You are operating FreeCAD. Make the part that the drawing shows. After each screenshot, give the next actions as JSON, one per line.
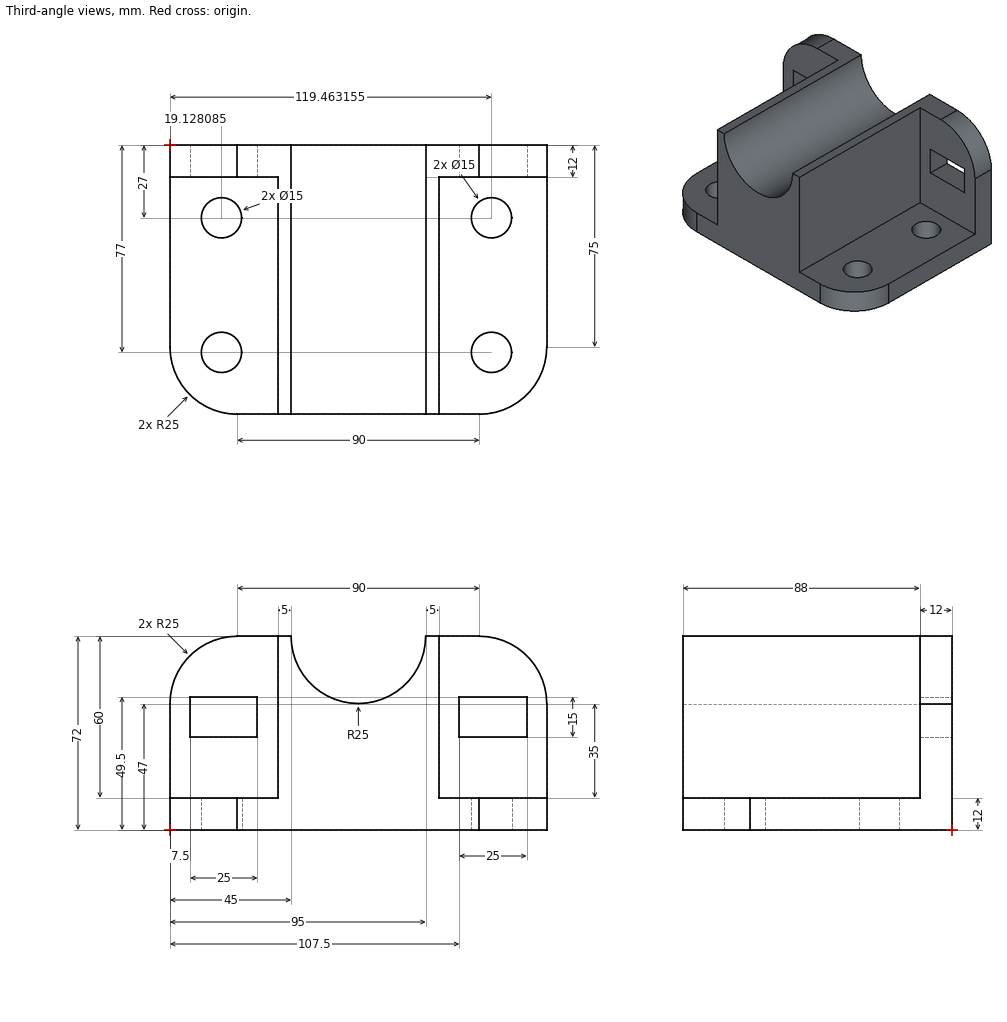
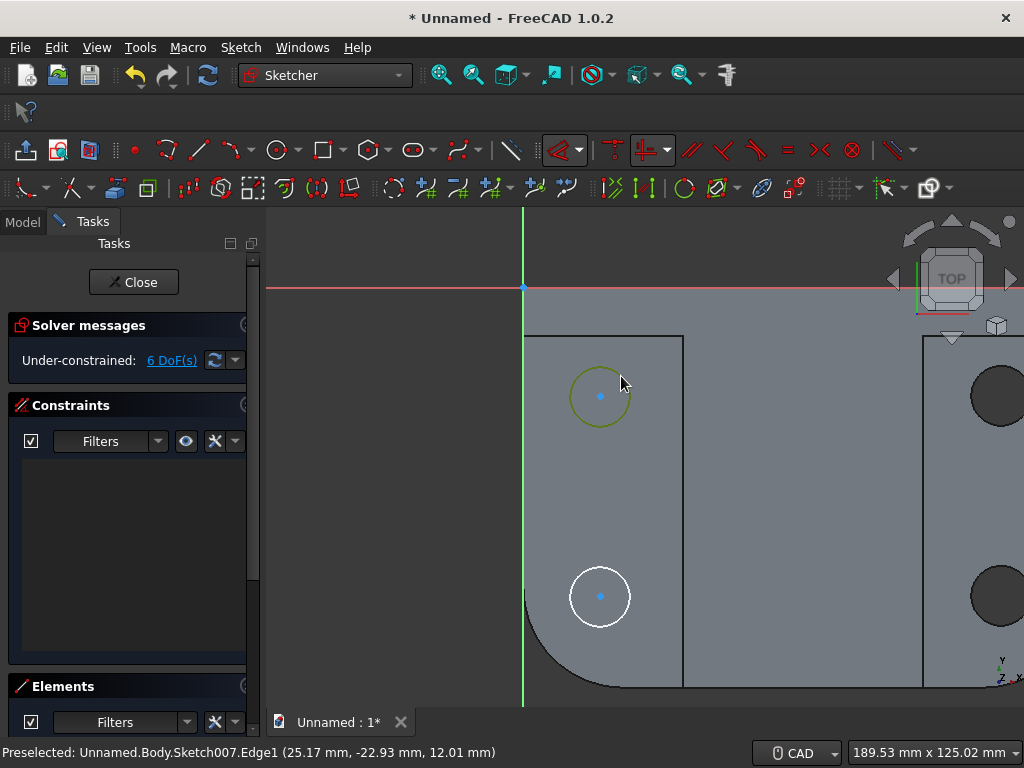
{"action": "left_click", "coordinate": [621, 576]}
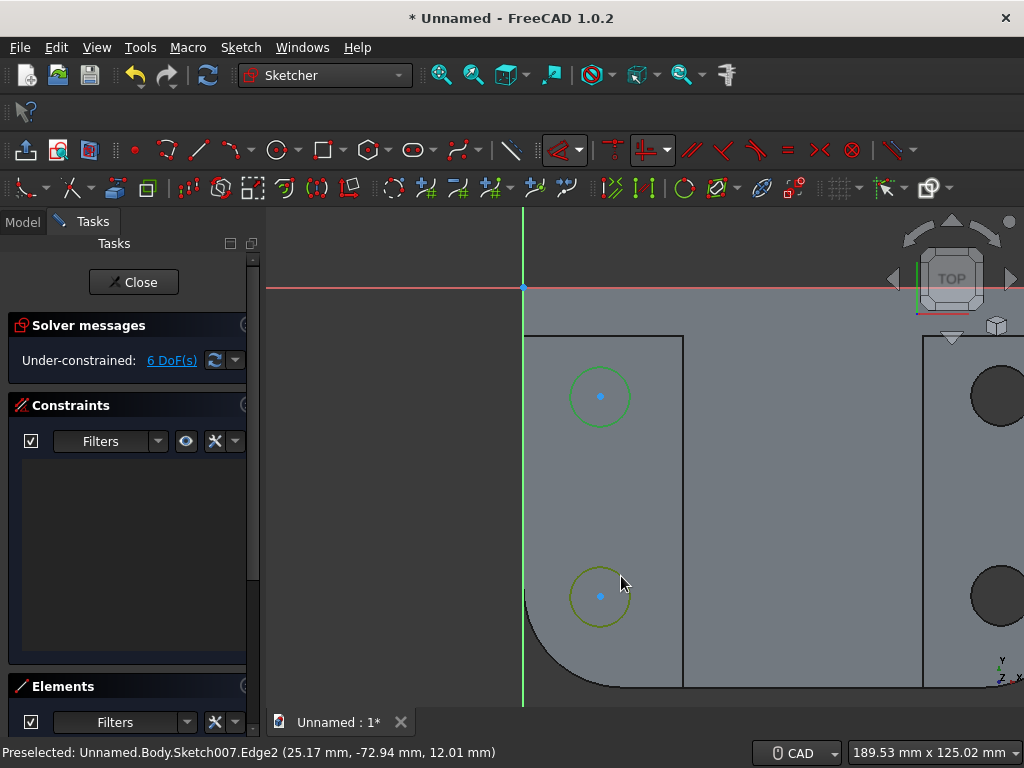
{"action": "left_click", "coordinate": [788, 150]}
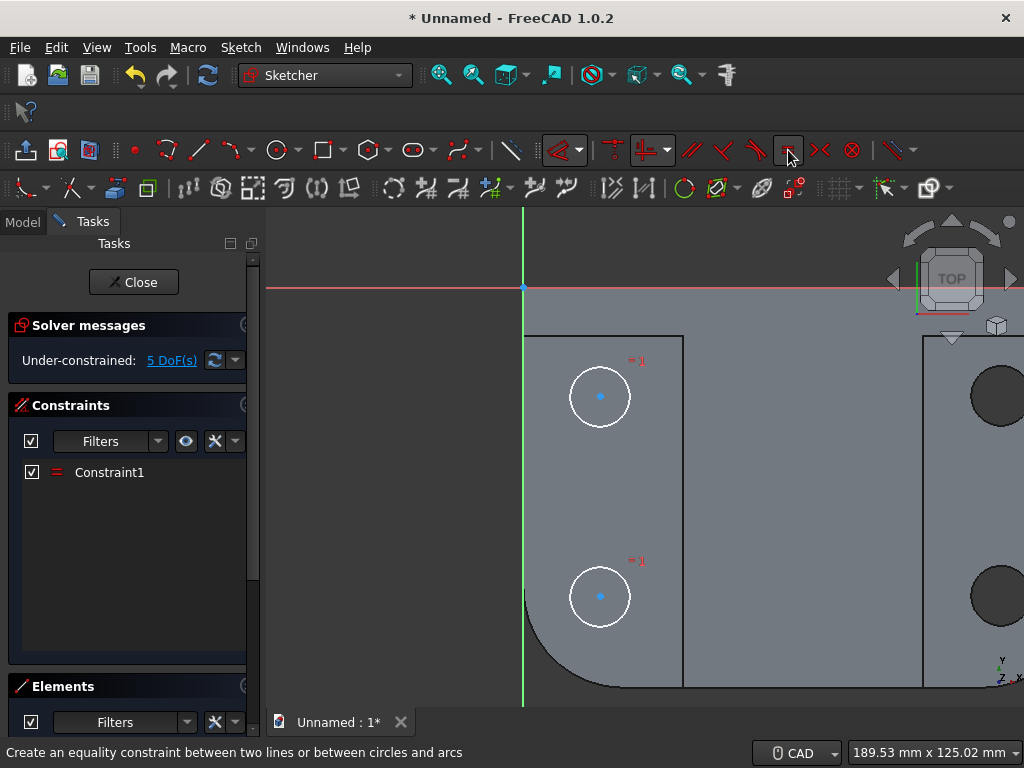
{"action": "left_click", "coordinate": [600, 397]}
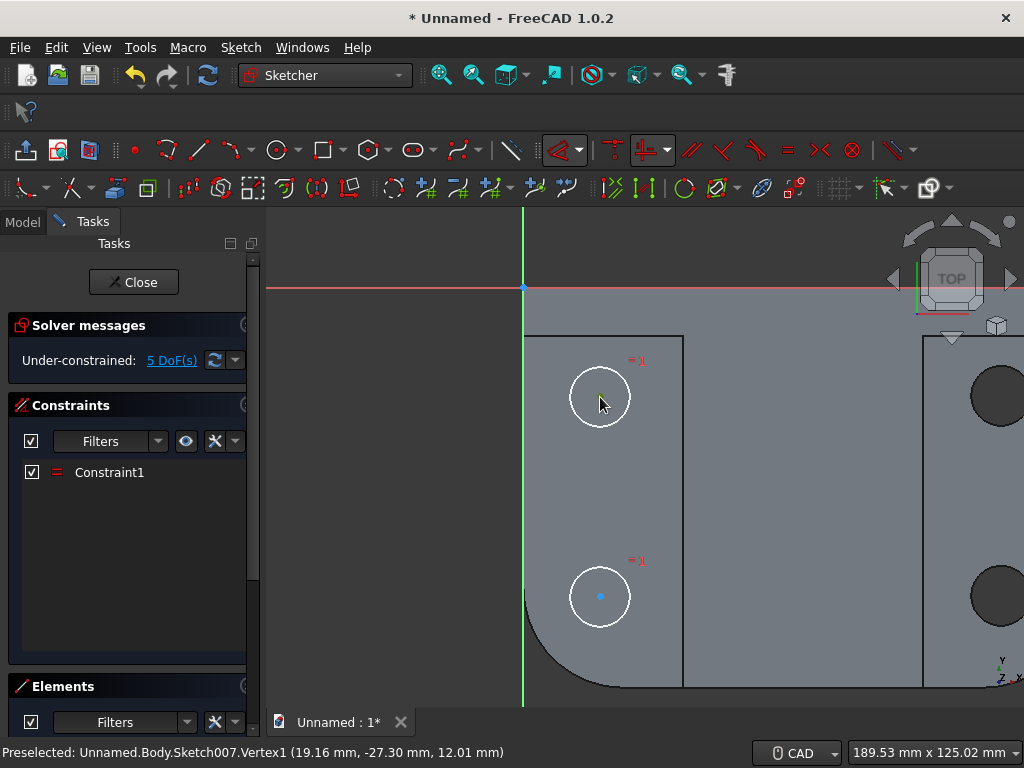
{"action": "left_click", "coordinate": [600, 597]}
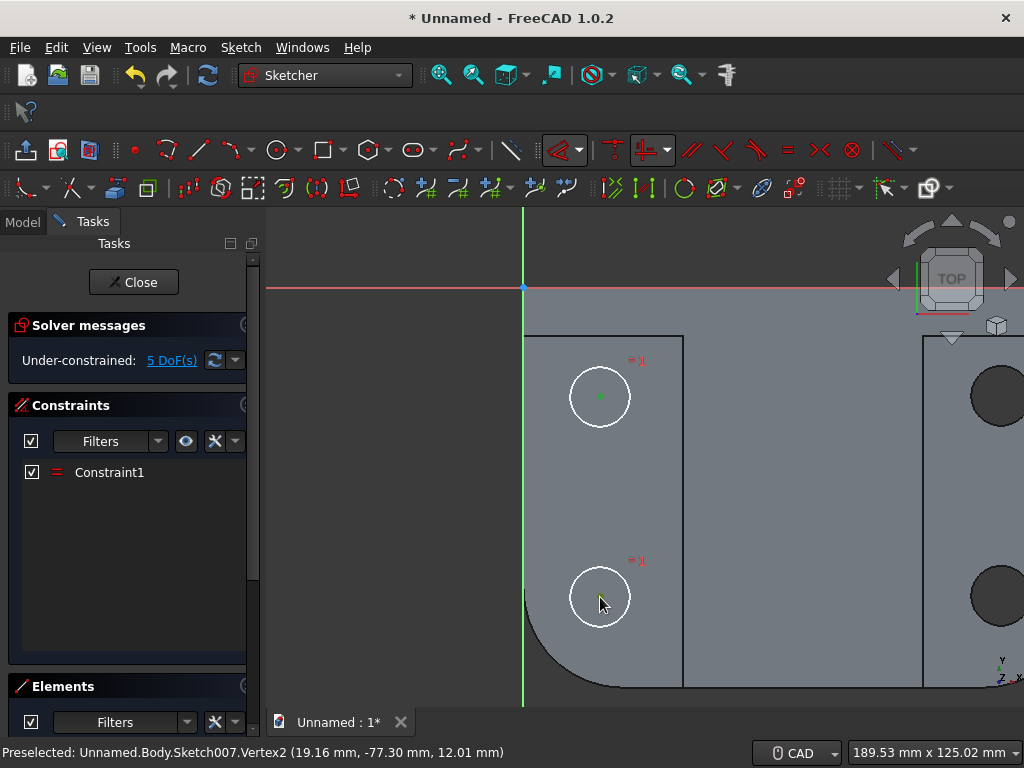
{"action": "key", "text": "v"}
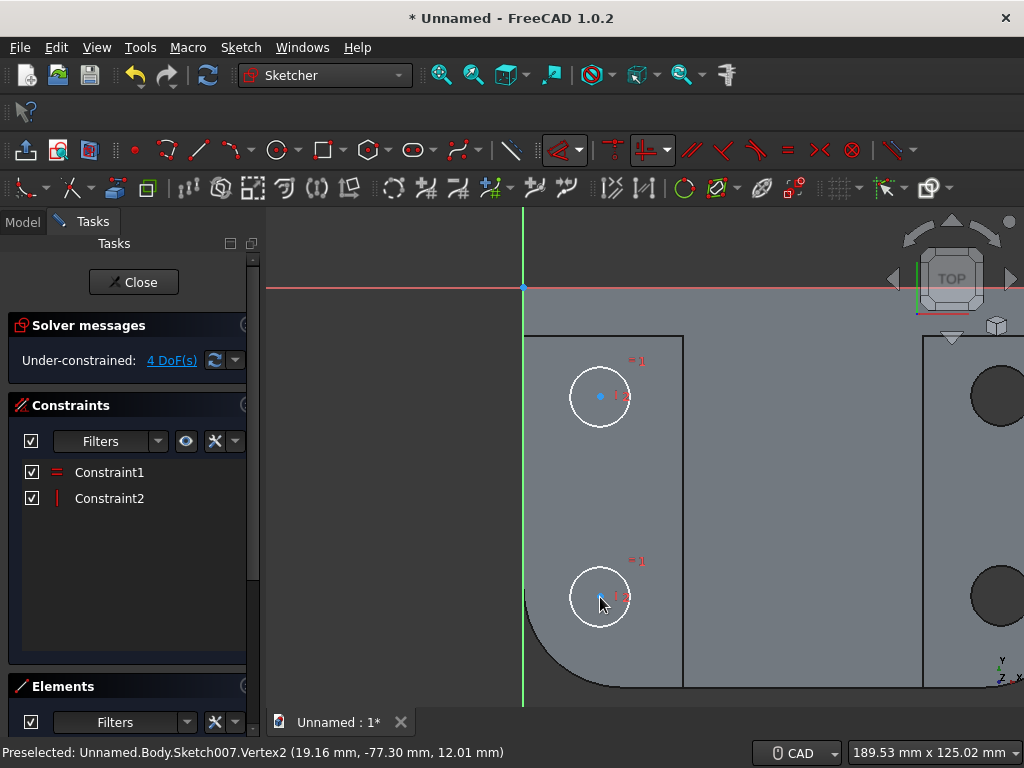
{"action": "left_click", "coordinate": [621, 376]}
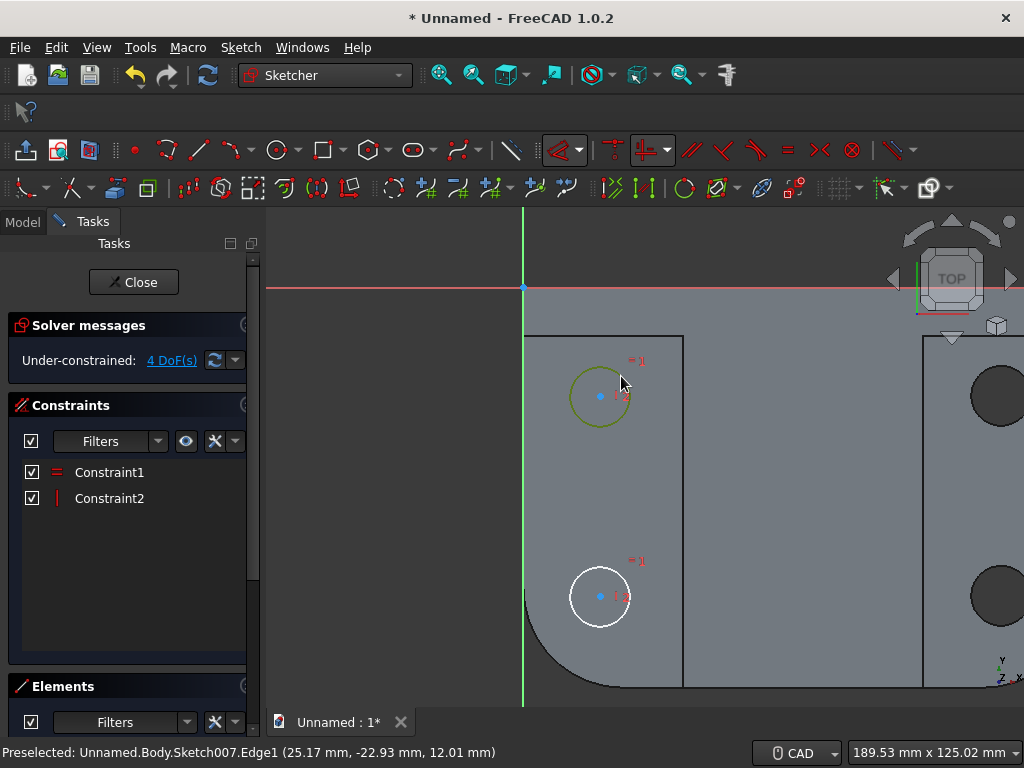
{"action": "key", "text": "k o"}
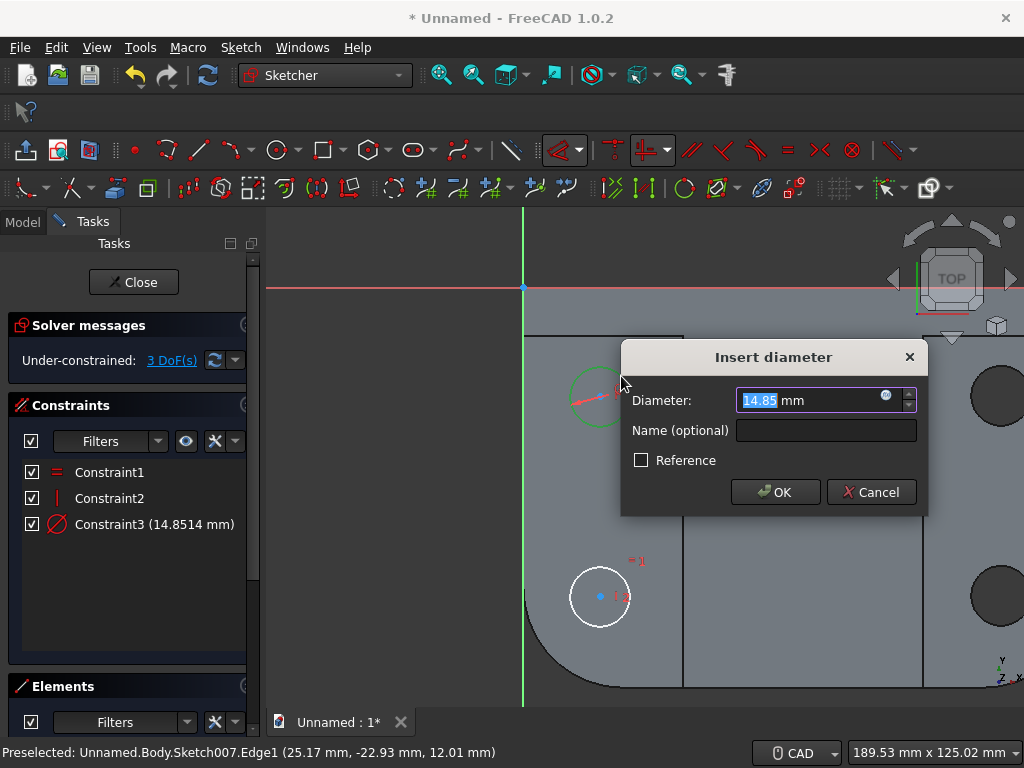
{"action": "type", "text": "15"}
{"action": "key", "text": "Return"}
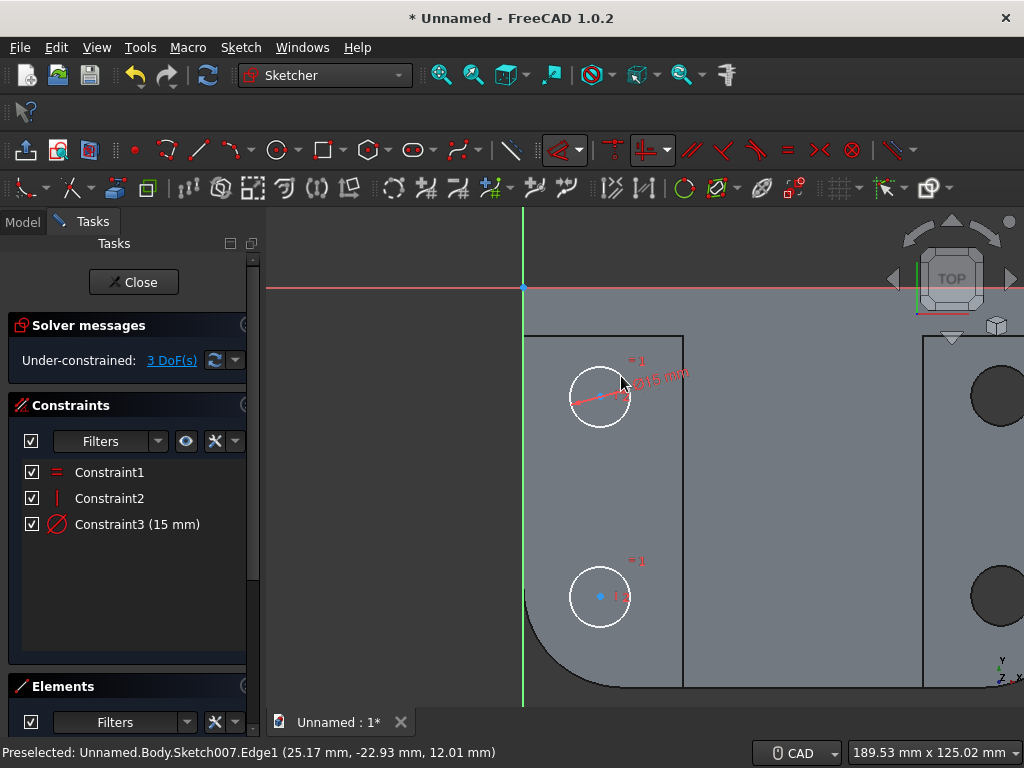
{"action": "left_click", "coordinate": [600, 397]}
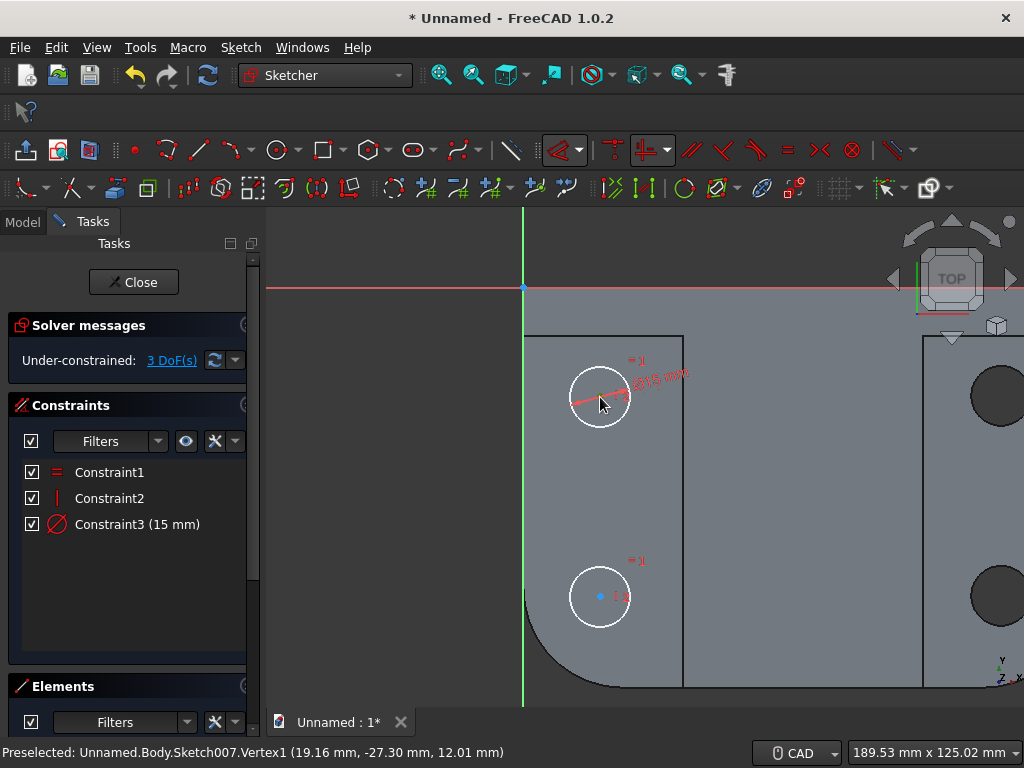
{"action": "key", "text": "i"}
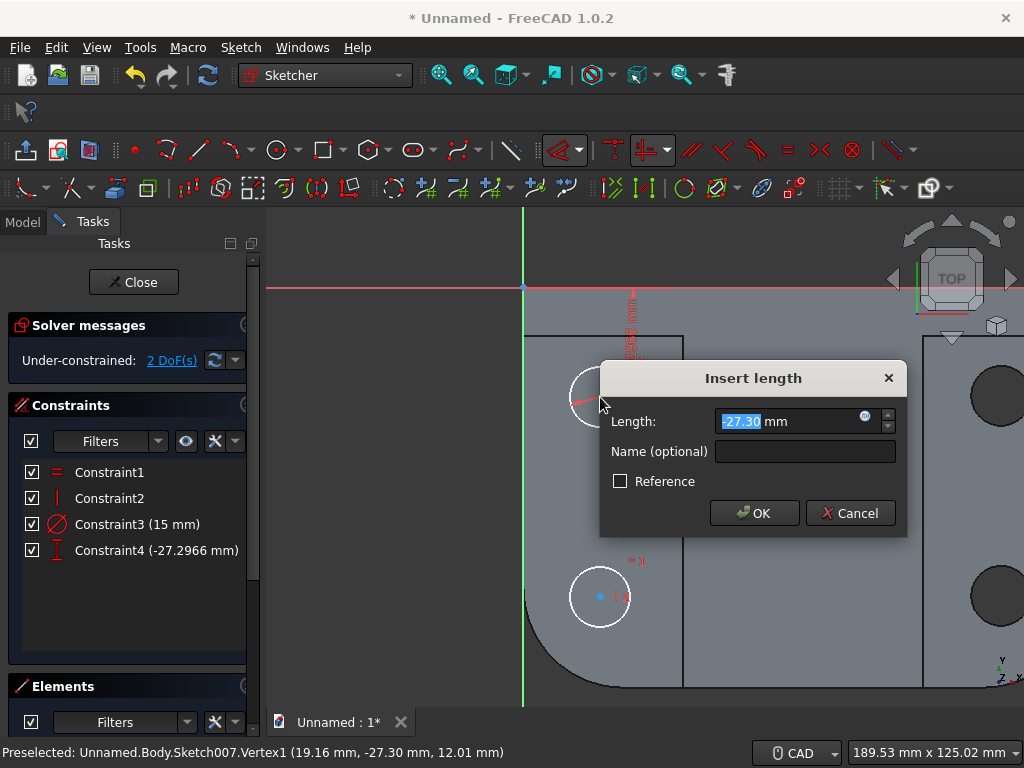
{"action": "type", "text": "-27"}
{"action": "key", "text": "Return"}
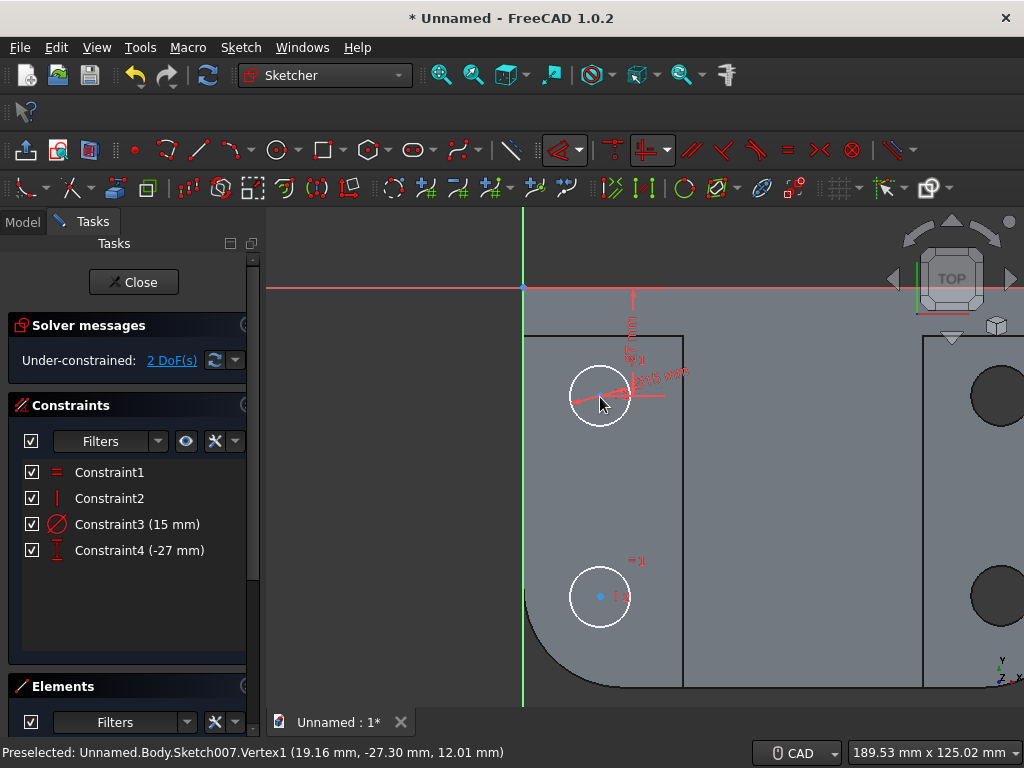
{"action": "left_click", "coordinate": [600, 597]}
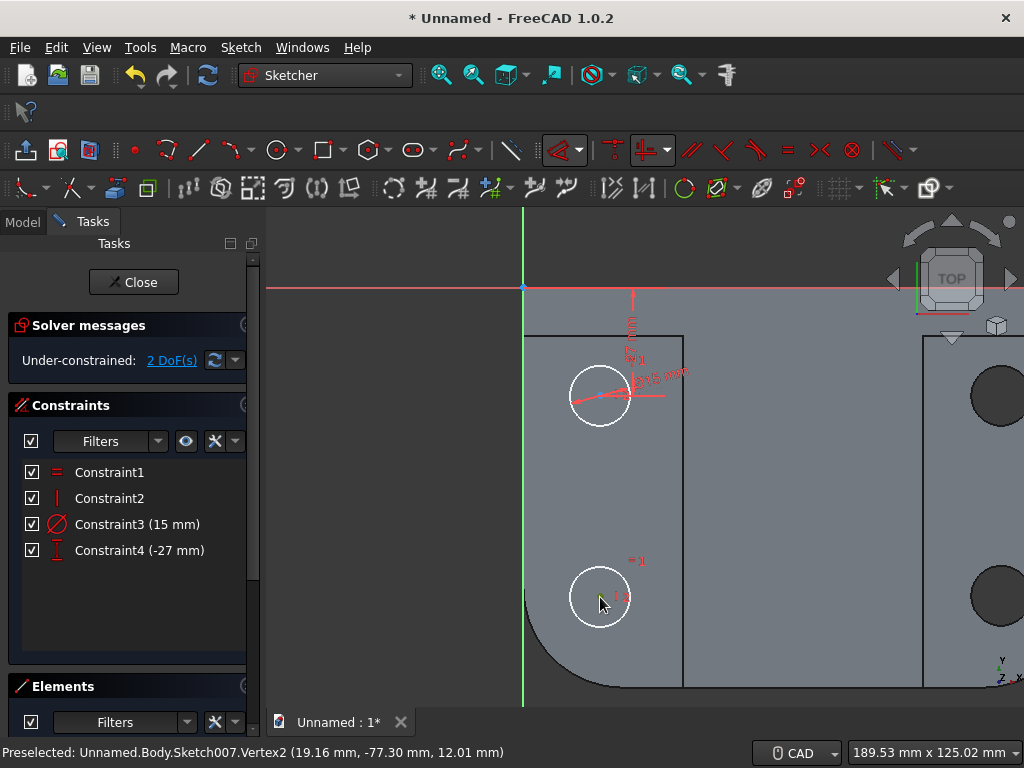
{"action": "left_click", "coordinate": [582, 150]}